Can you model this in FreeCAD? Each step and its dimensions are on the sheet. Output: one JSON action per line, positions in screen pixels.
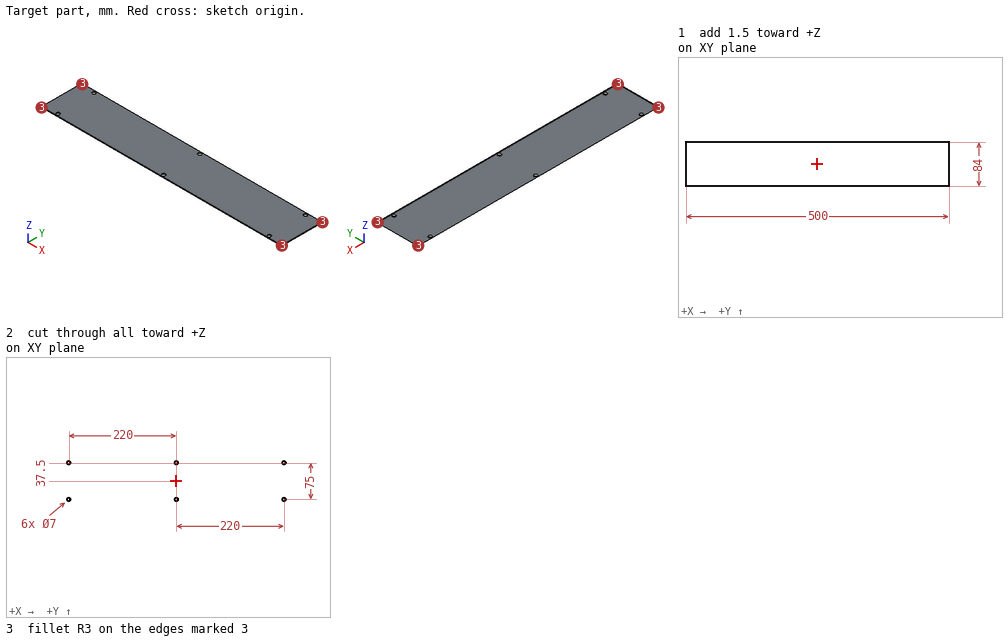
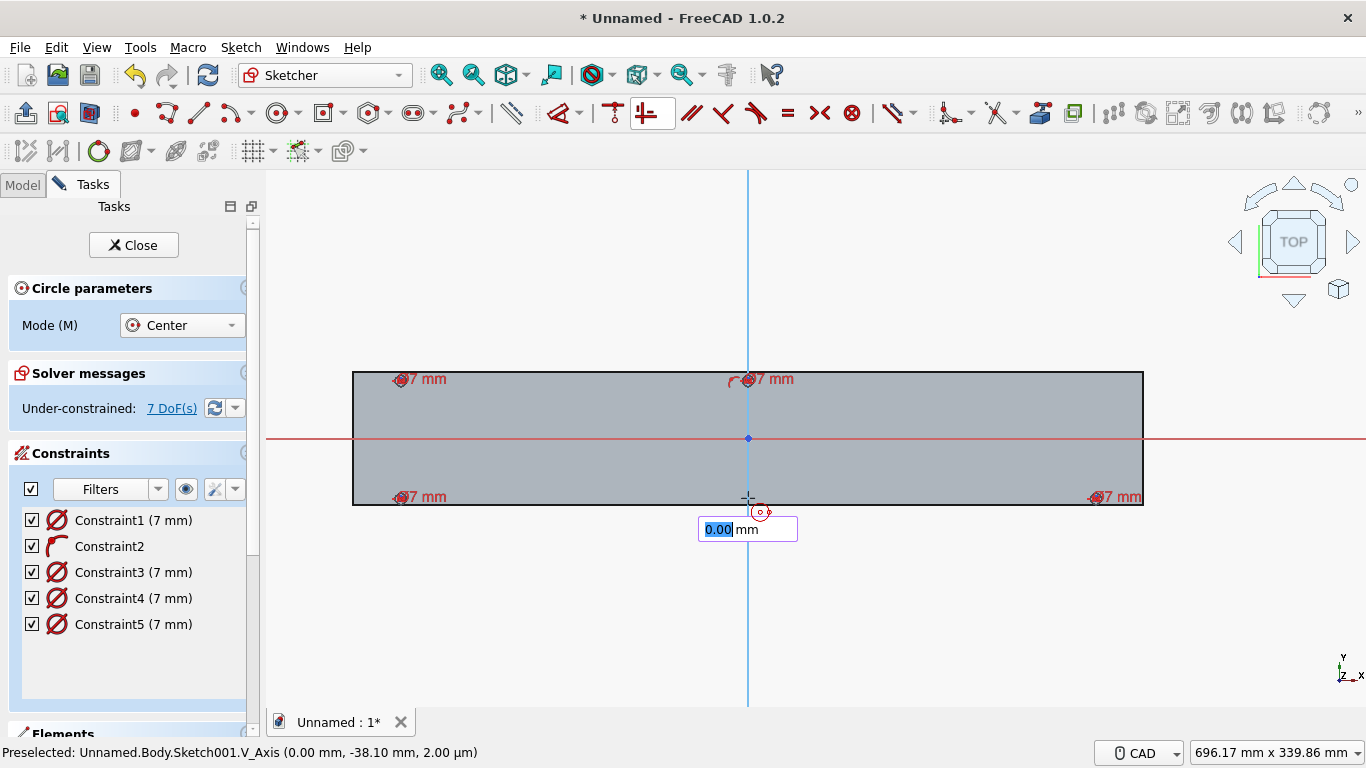
{"action": "scroll", "coordinate": [753, 496], "scroll_direction": "up", "scroll_amount": 6}
{"action": "mouse_move", "coordinate": [753, 495]}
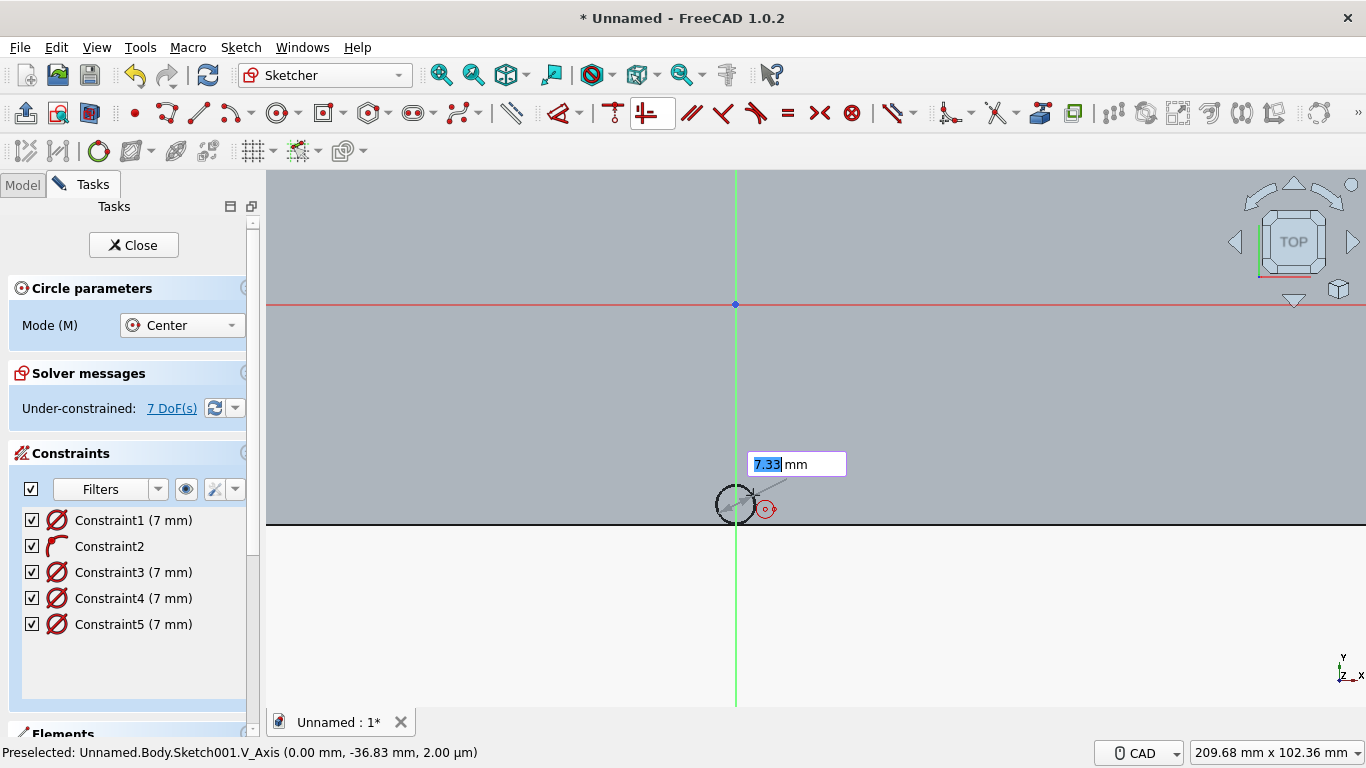
{"action": "type", "text": "7"}
{"action": "key", "text": "Return"}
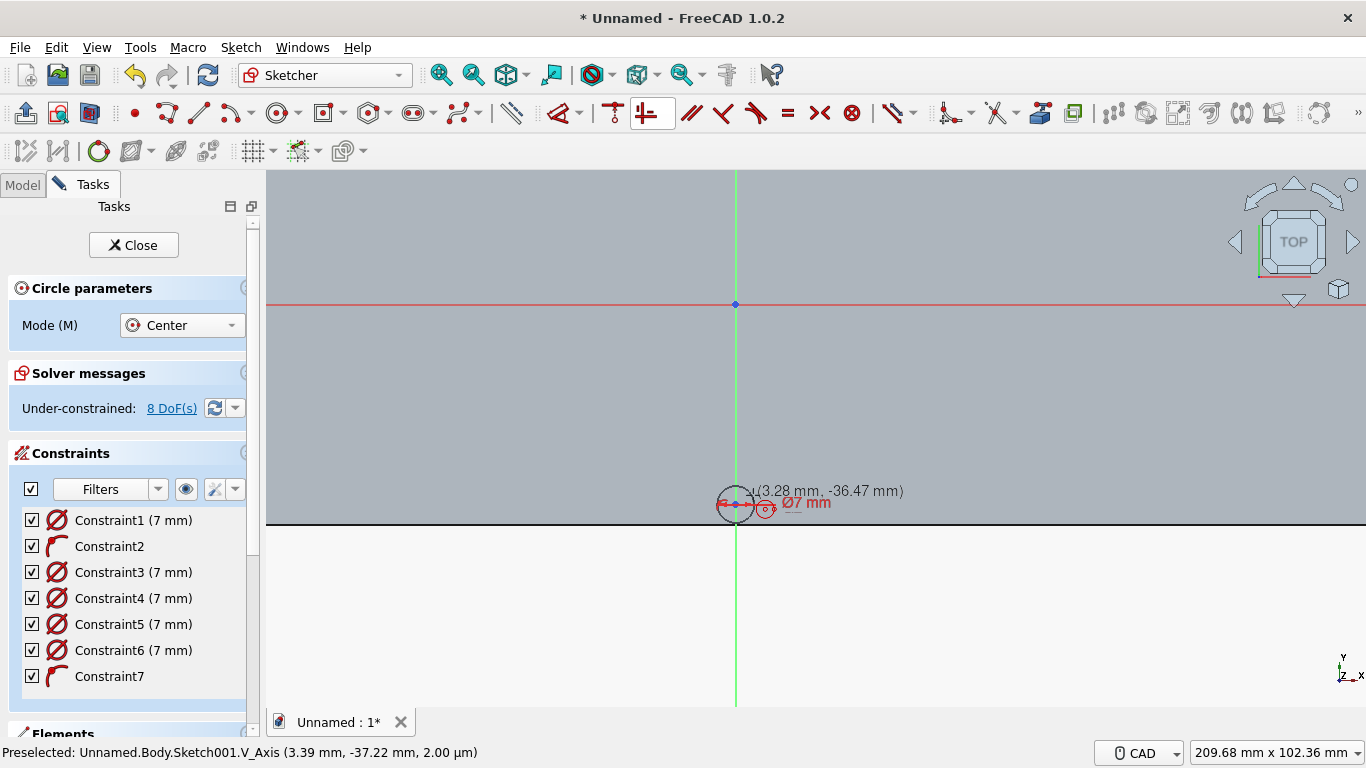
{"action": "scroll", "coordinate": [753, 496], "scroll_direction": "down", "scroll_amount": 6}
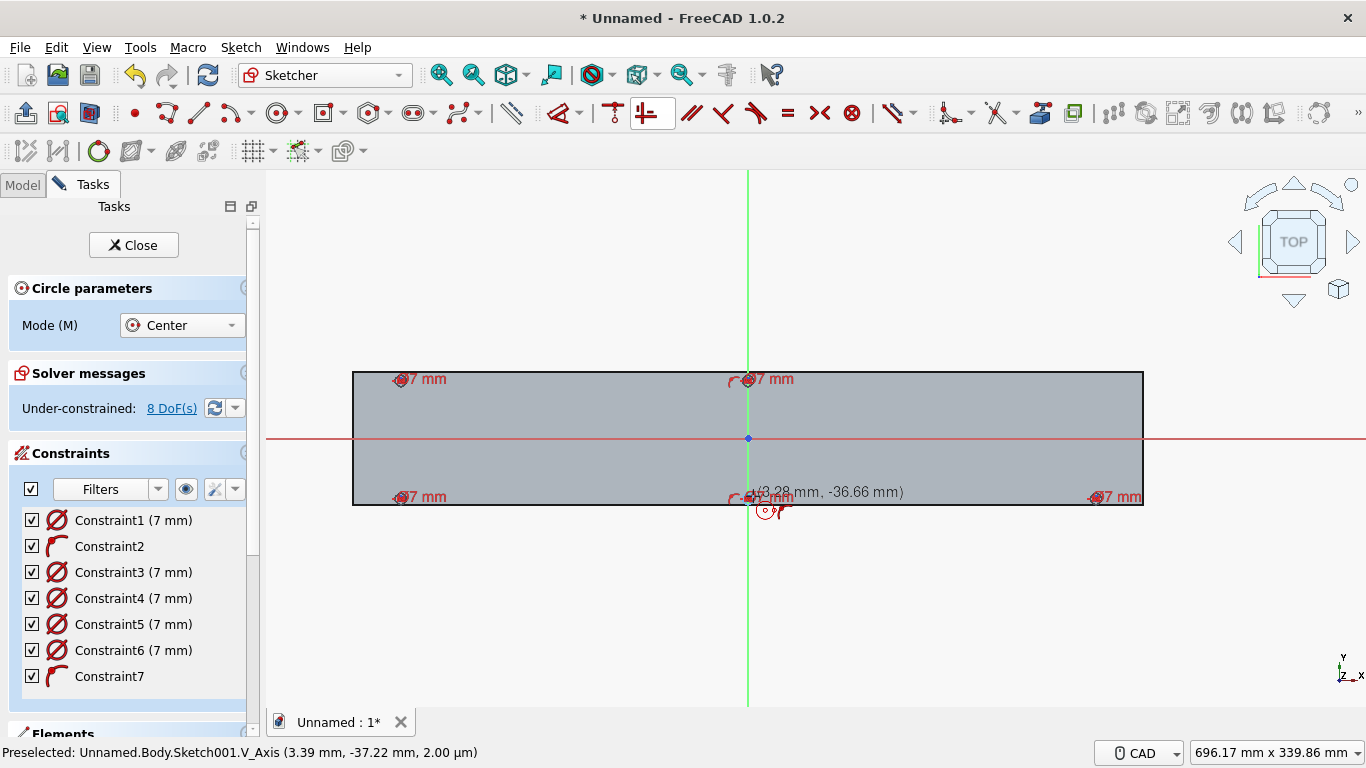
{"action": "scroll", "coordinate": [1096, 380], "scroll_direction": "up", "scroll_amount": 8}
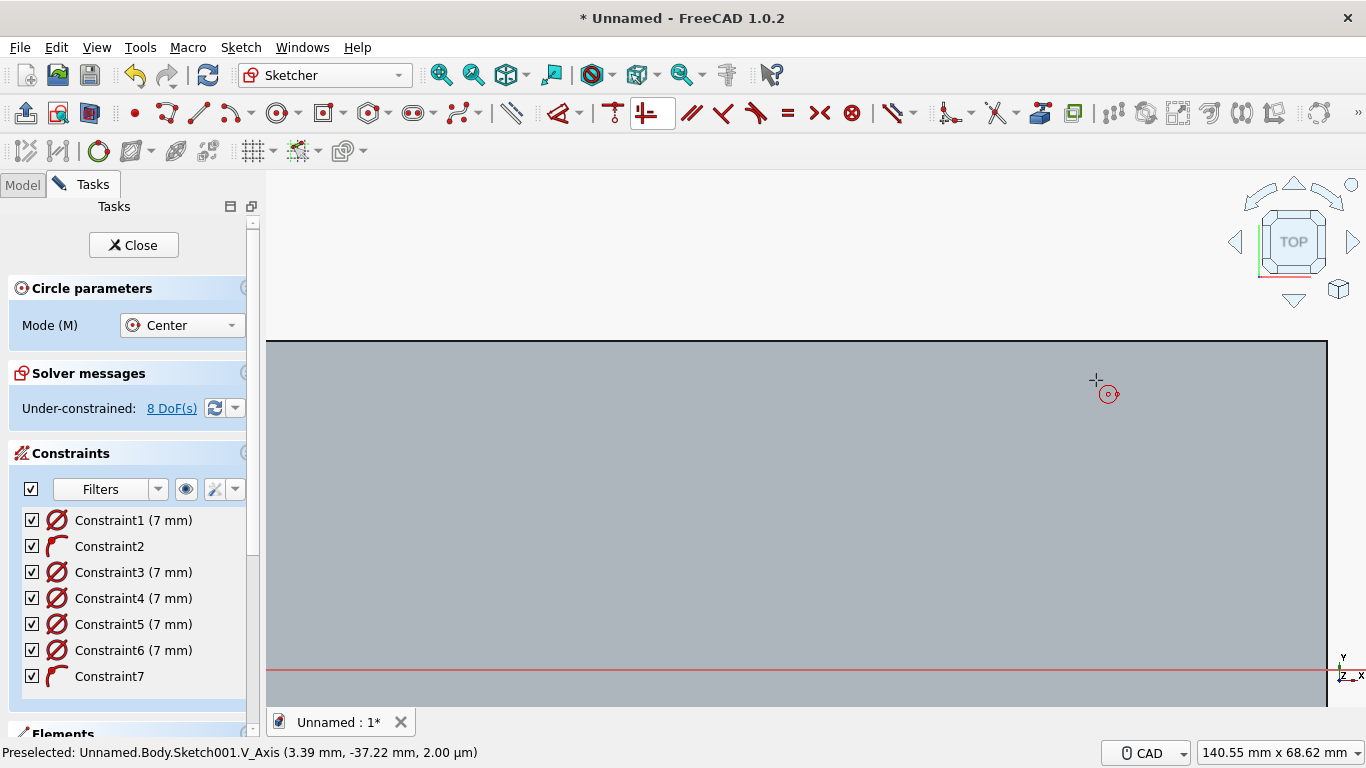
{"action": "scroll", "coordinate": [1096, 380], "scroll_direction": "down", "scroll_amount": 8}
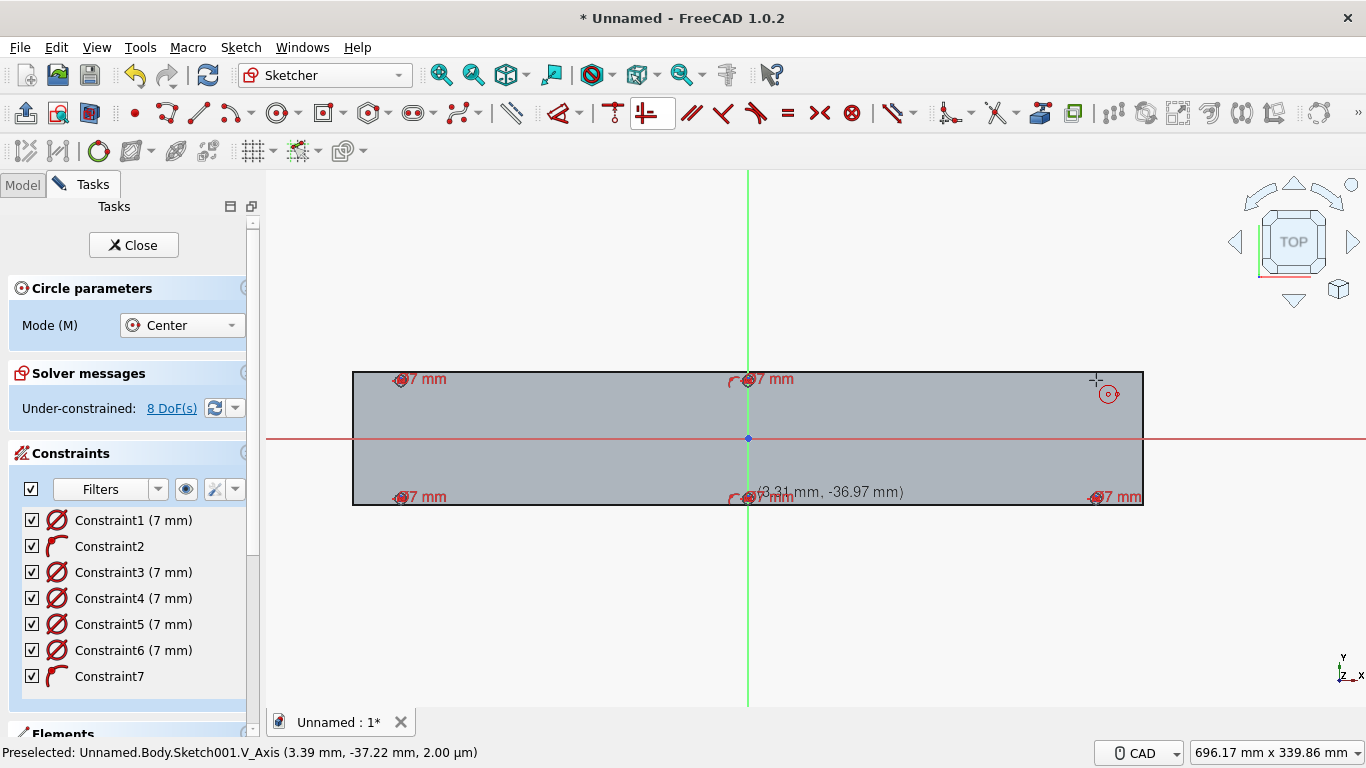
{"action": "left_click", "coordinate": [1096, 380]}
{"action": "mouse_move", "coordinate": [1100, 376]}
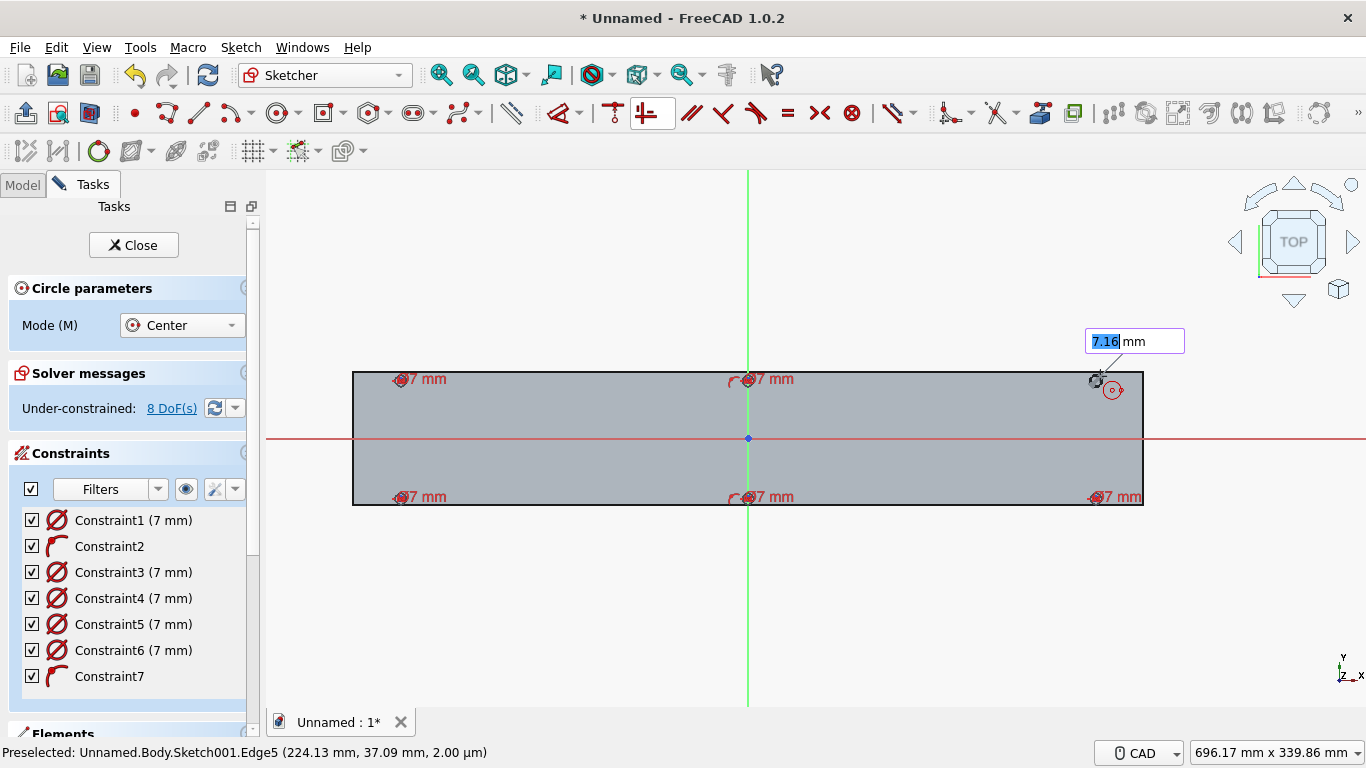
{"action": "type", "text": "7"}
{"action": "key", "text": "Return"}
{"action": "key", "text": "Escape"}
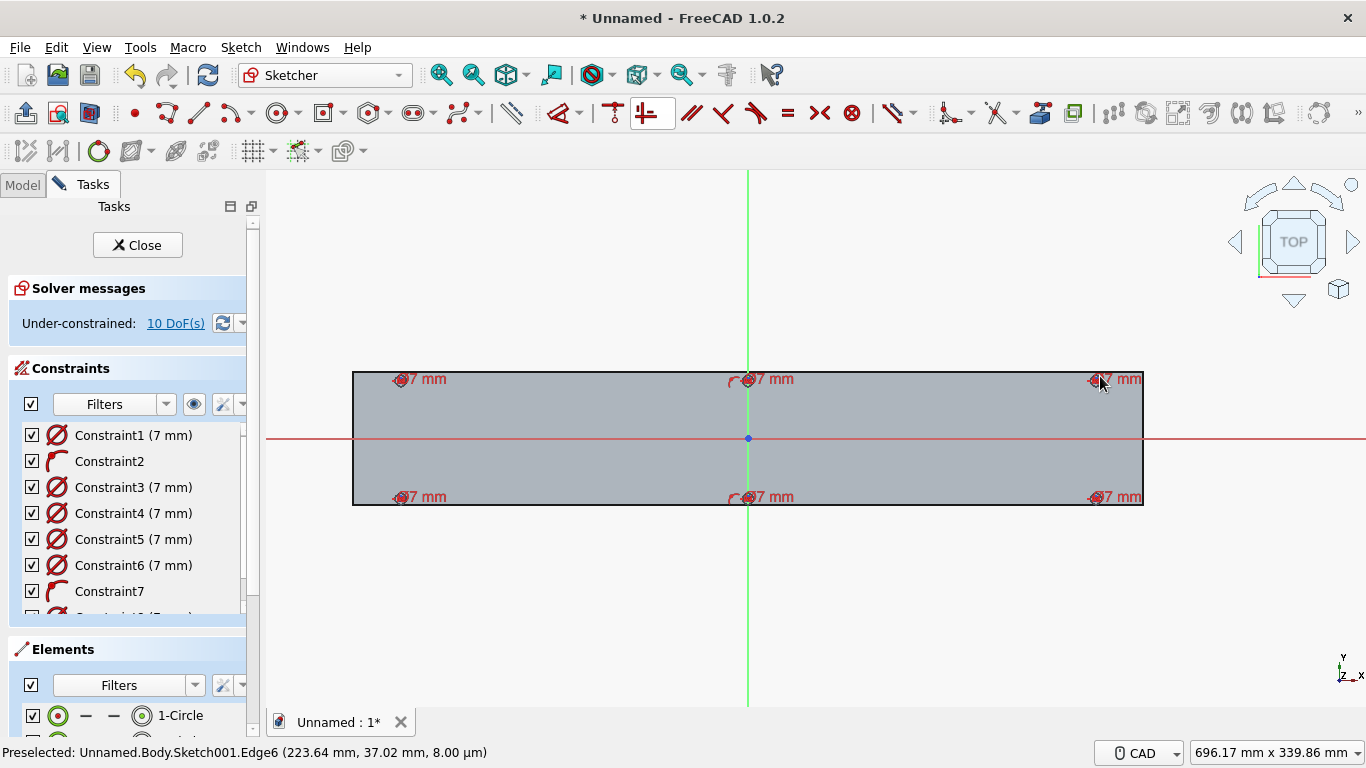
{"action": "left_click", "coordinate": [748, 381]}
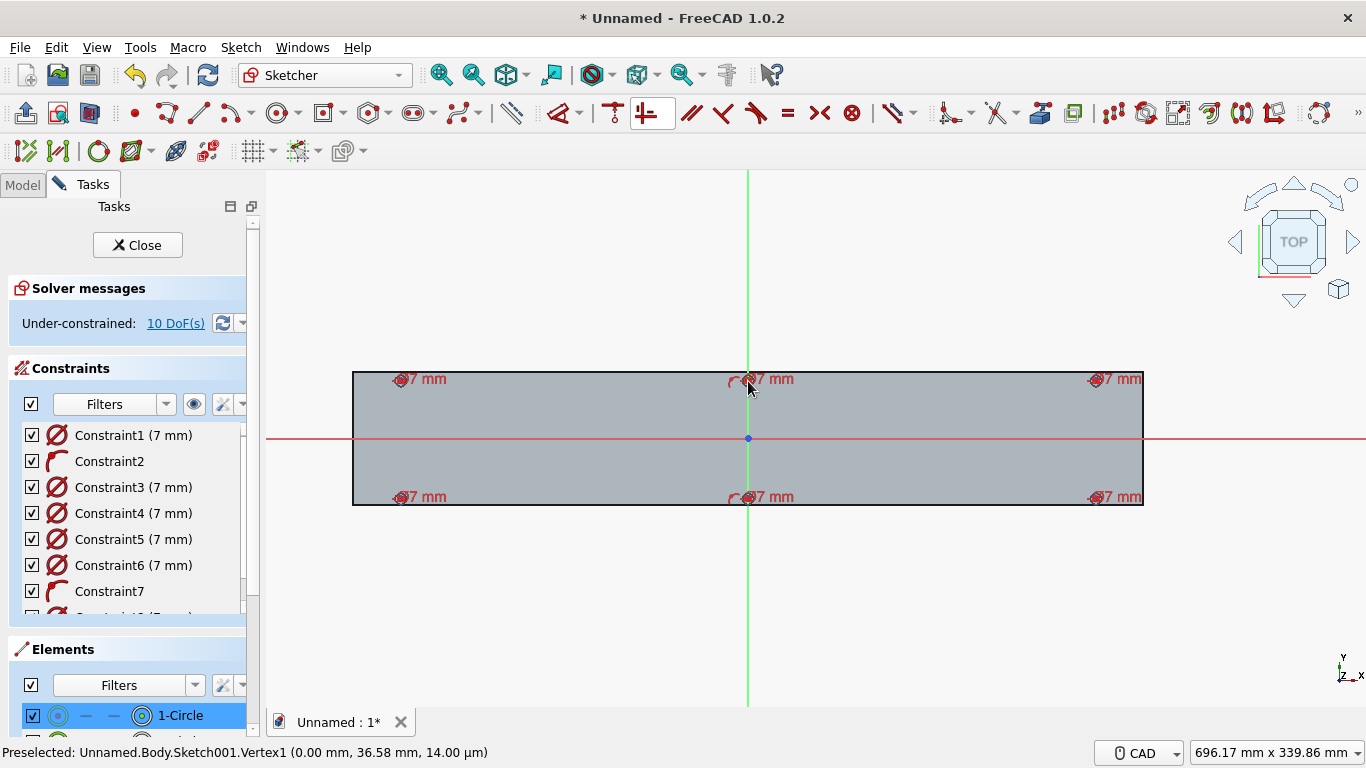
{"action": "left_click", "coordinate": [401, 381]}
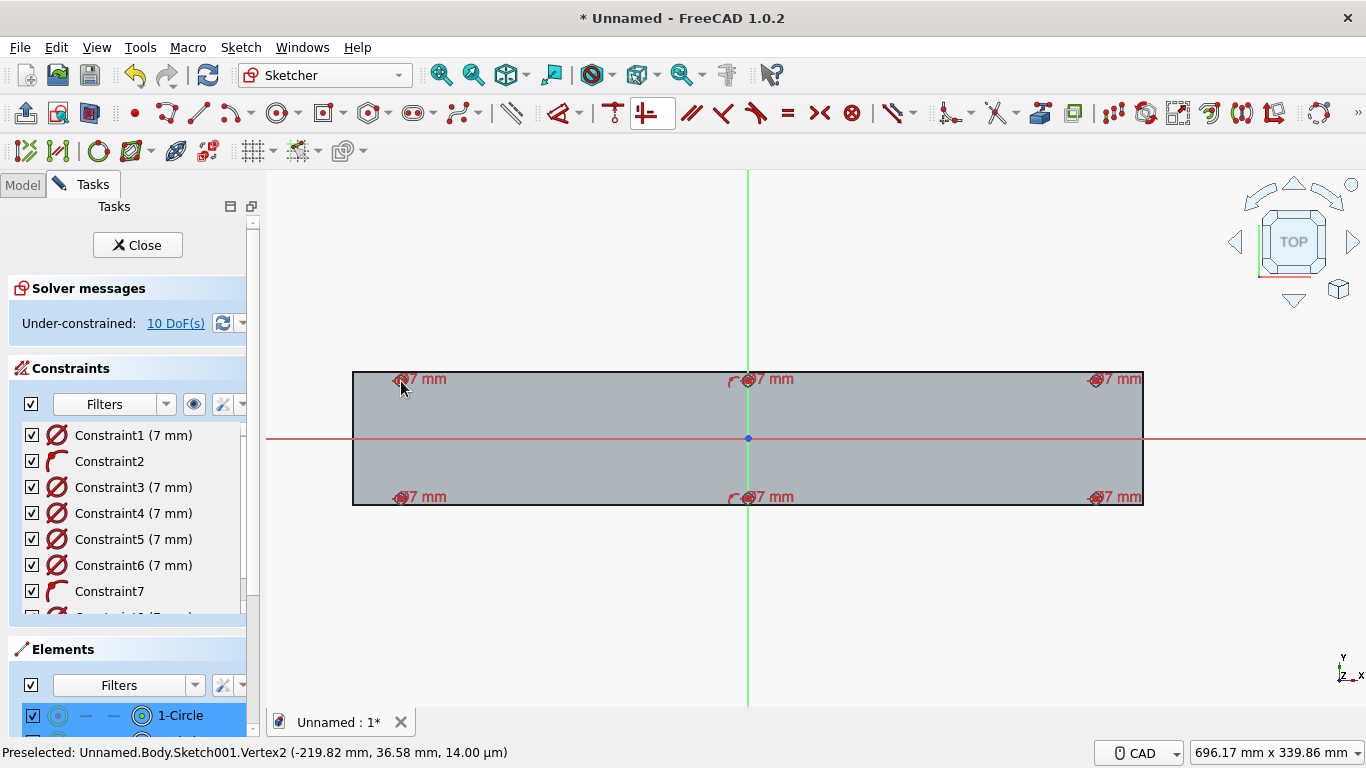
{"action": "key", "text": "h"}